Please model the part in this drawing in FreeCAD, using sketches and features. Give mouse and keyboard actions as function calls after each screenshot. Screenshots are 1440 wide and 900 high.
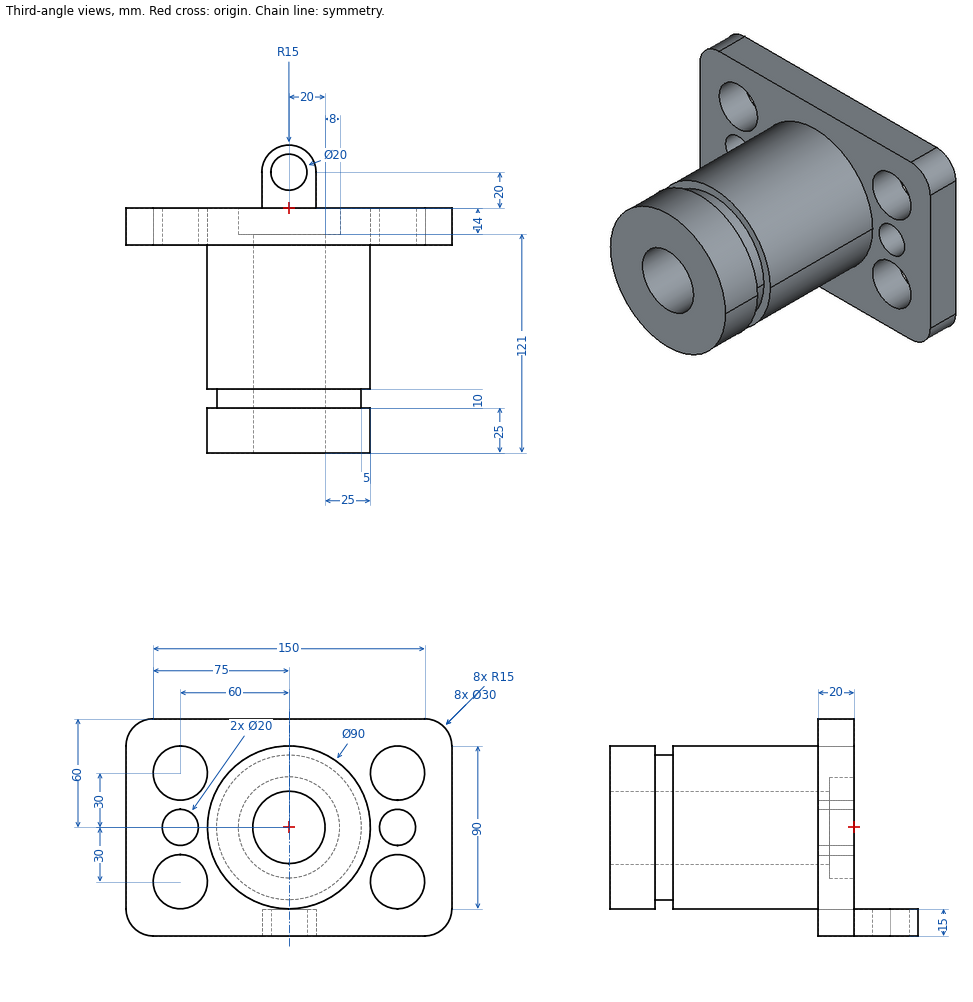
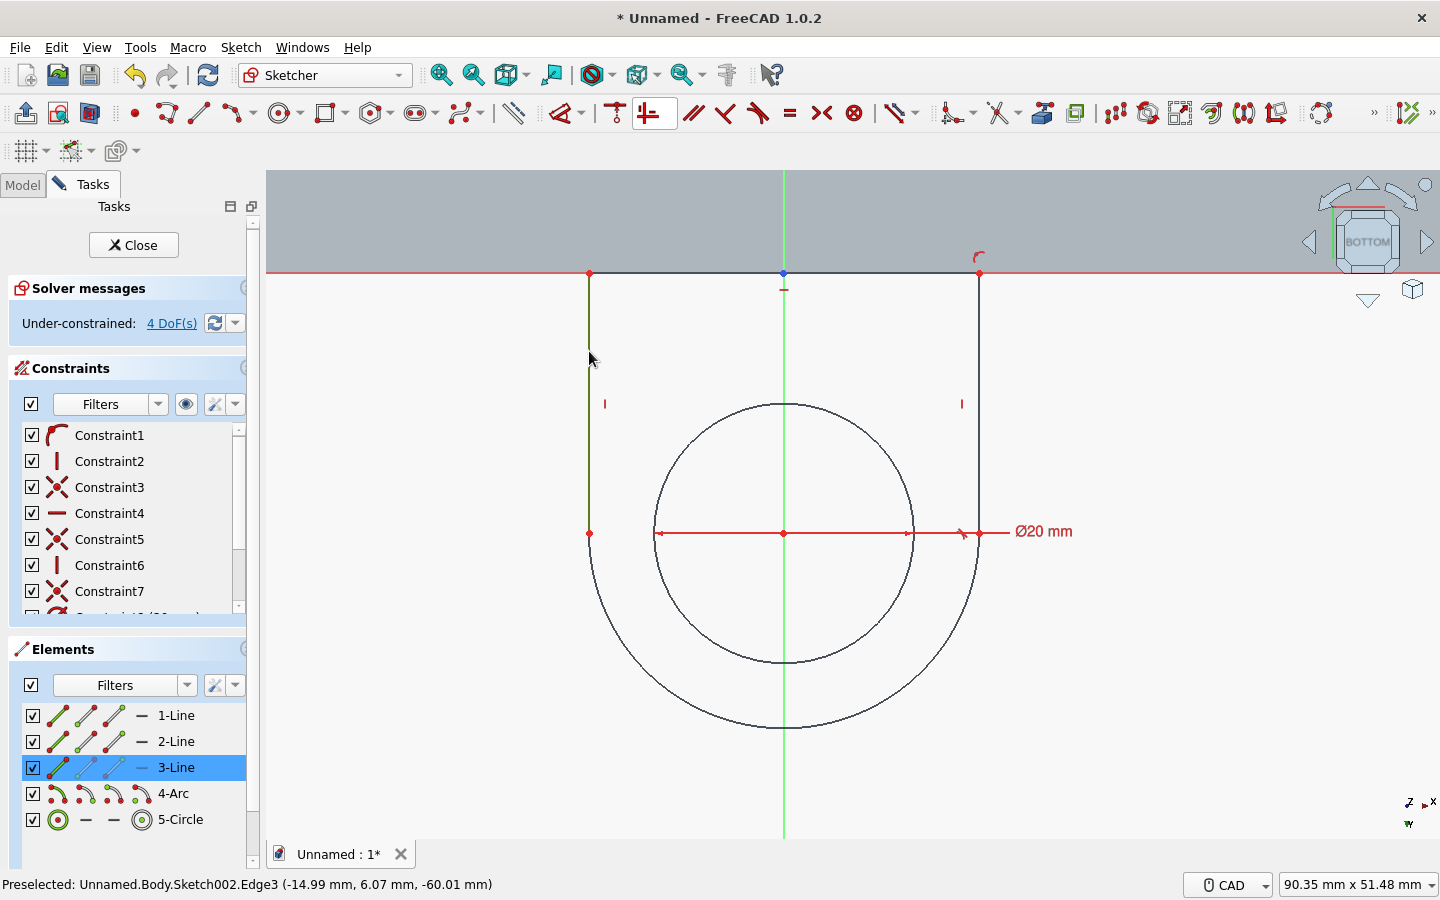
click(670, 691)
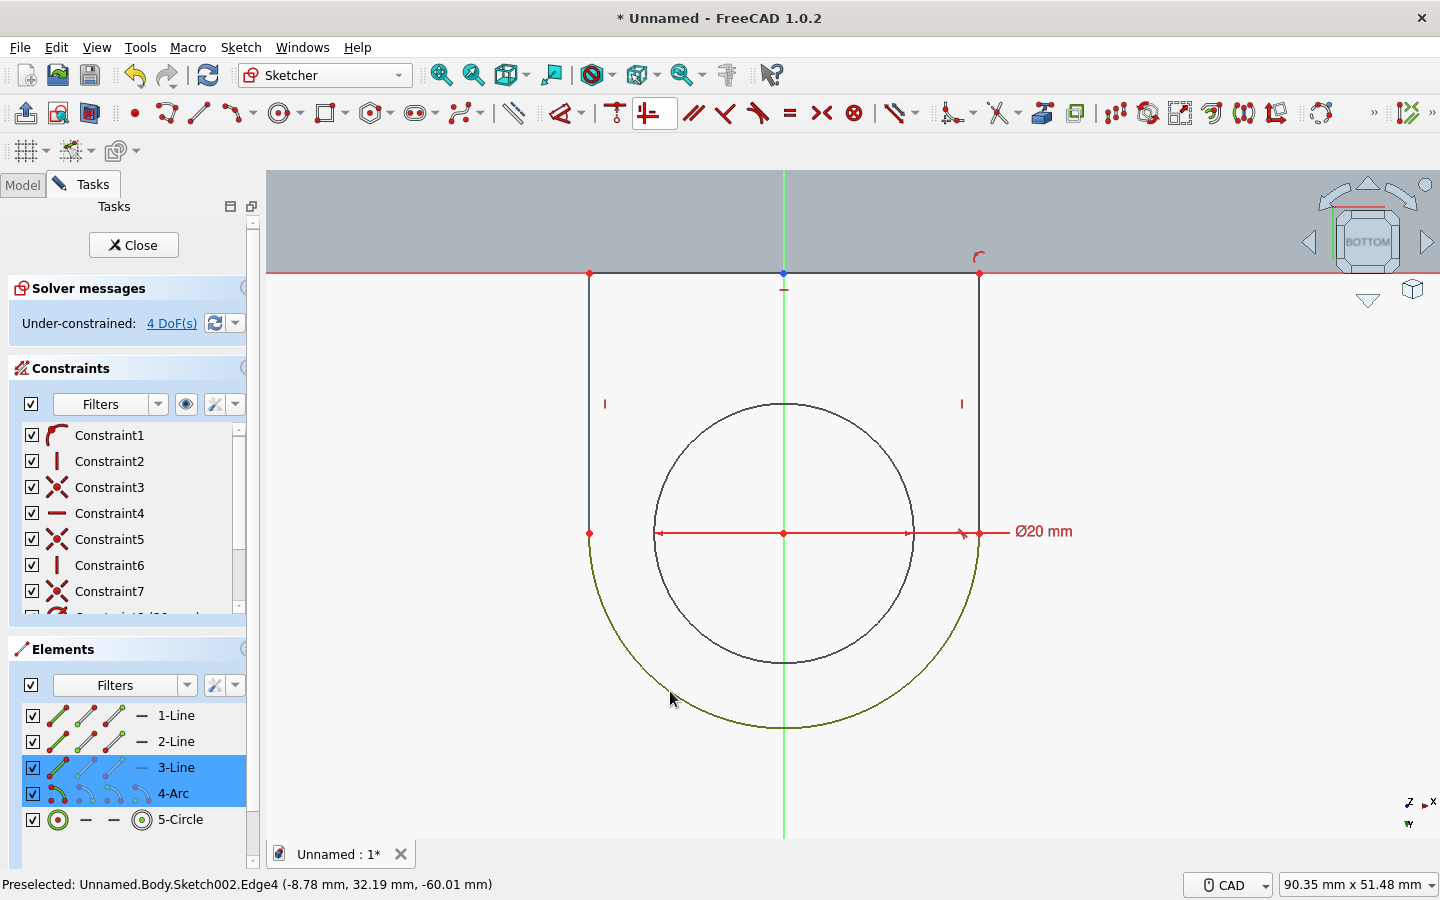
click(758, 114)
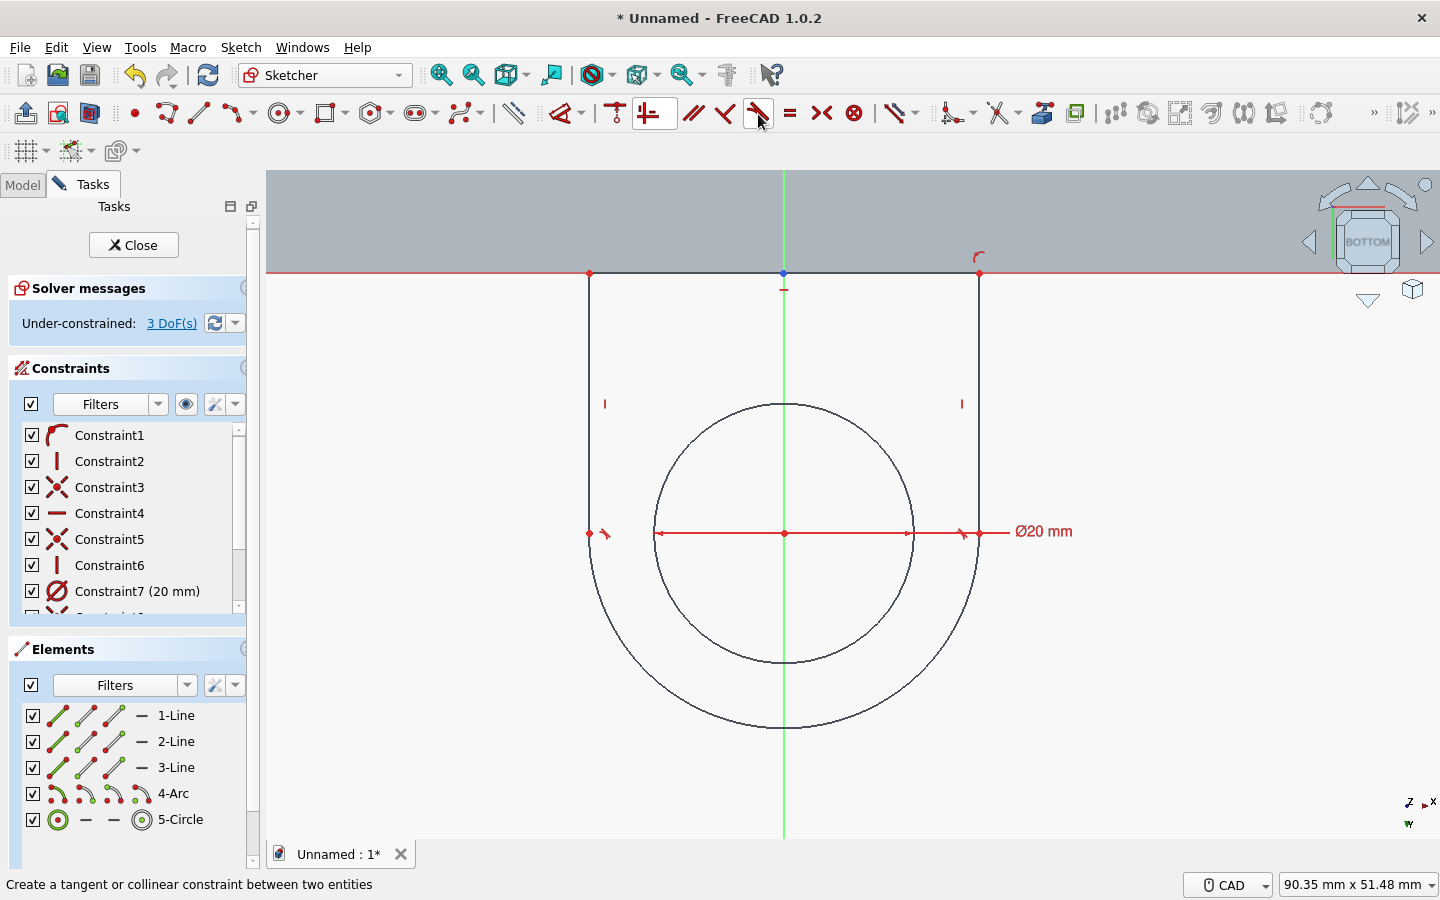
click(784, 533)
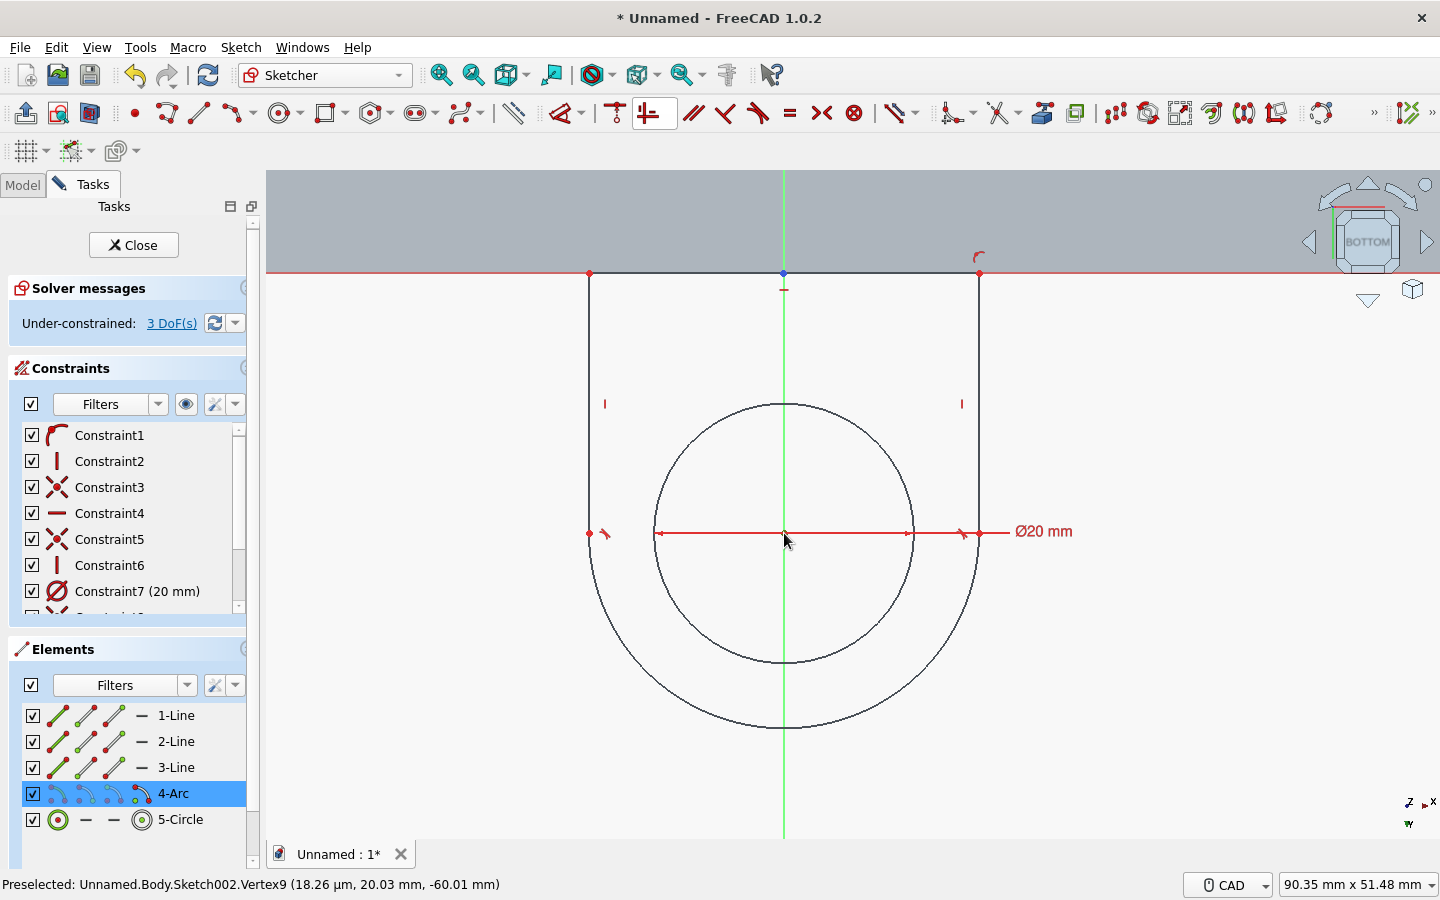
click(784, 767)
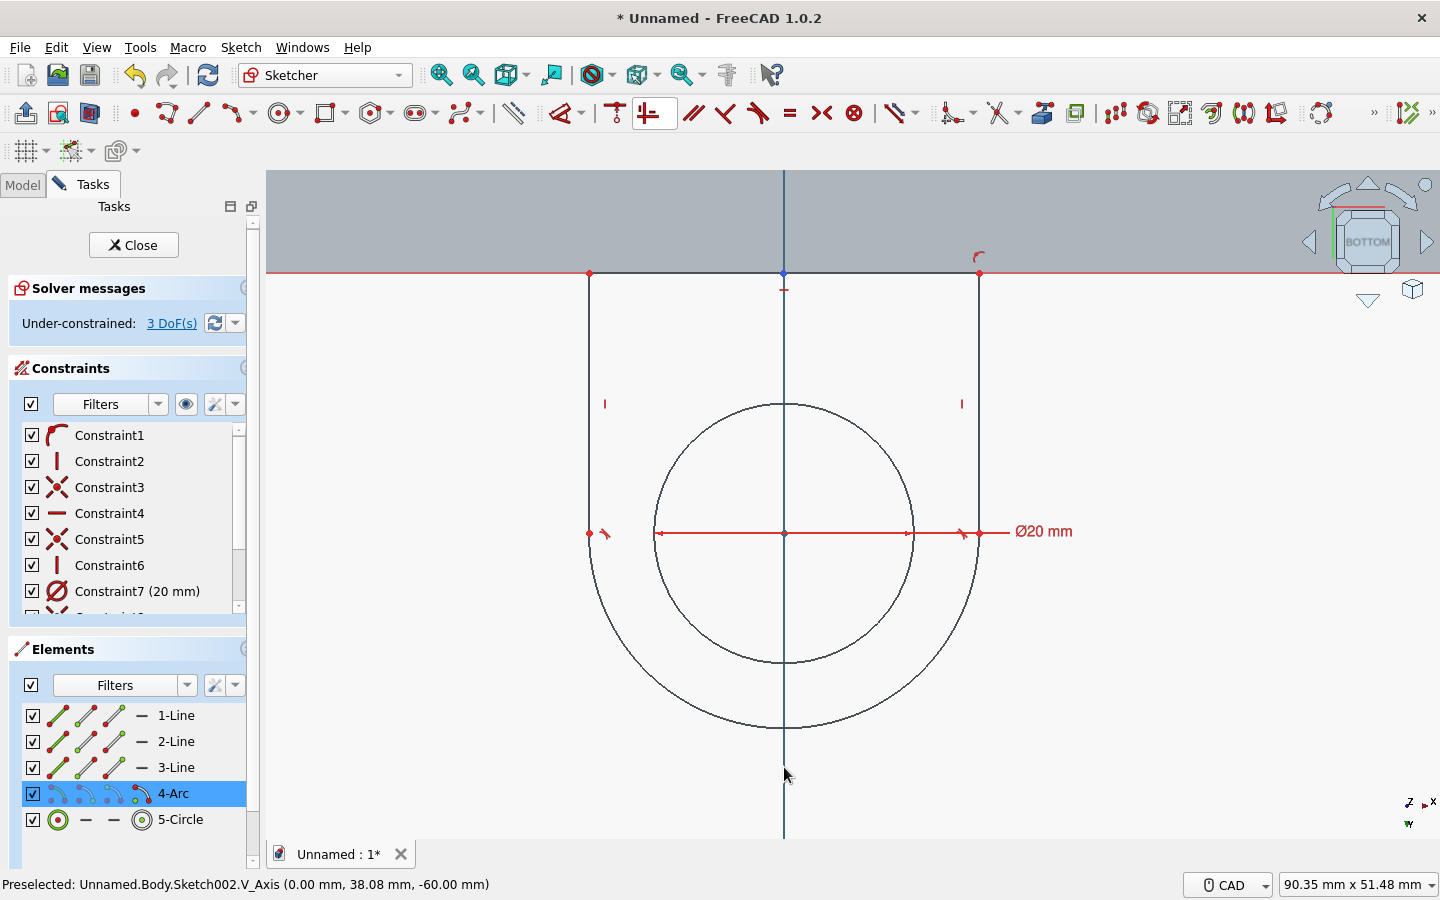
click(616, 114)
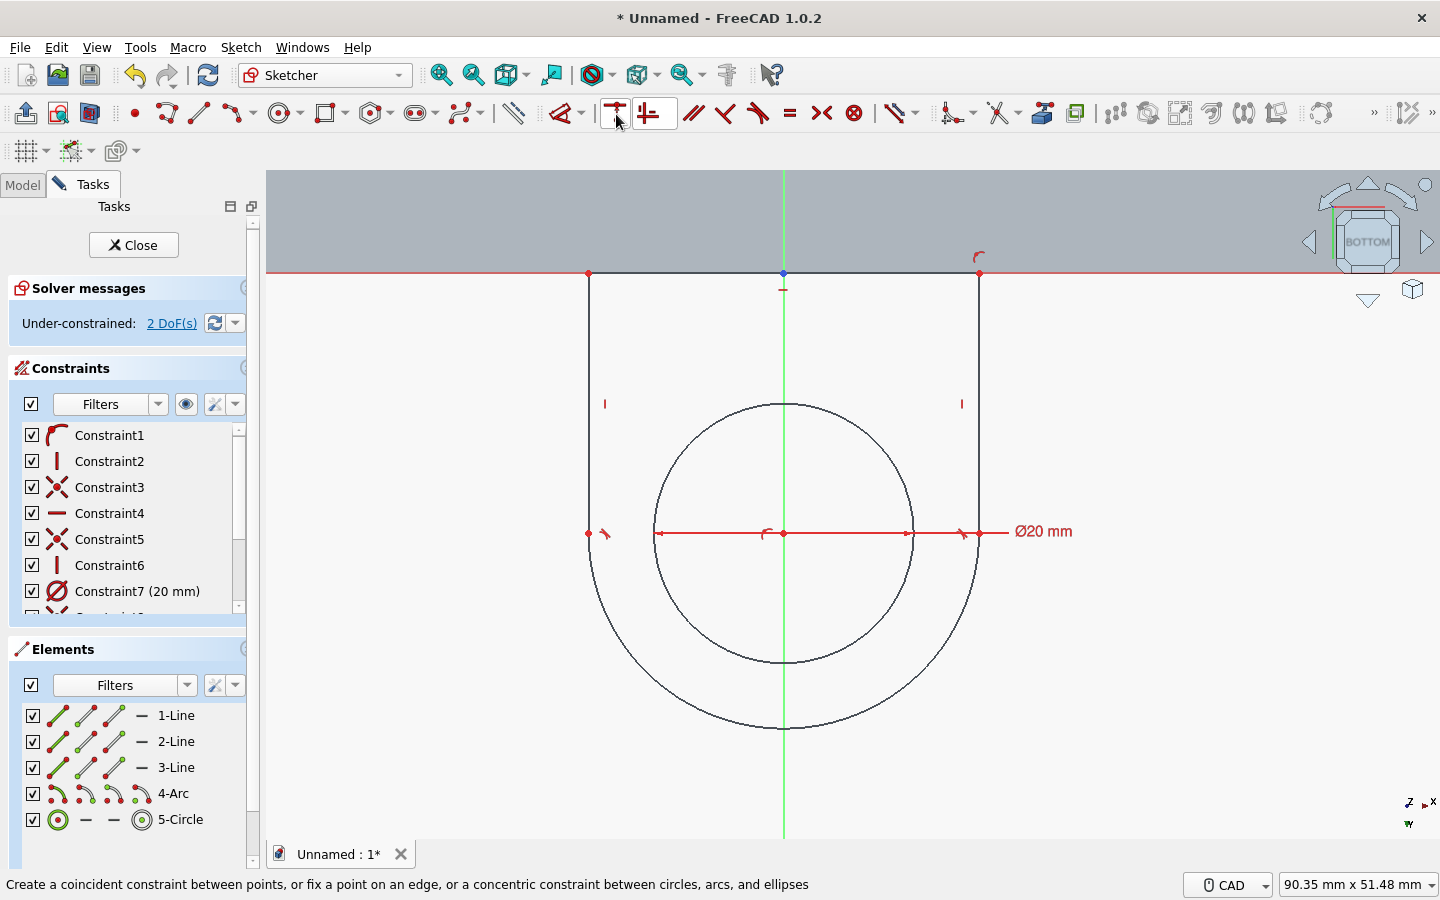
click(560, 114)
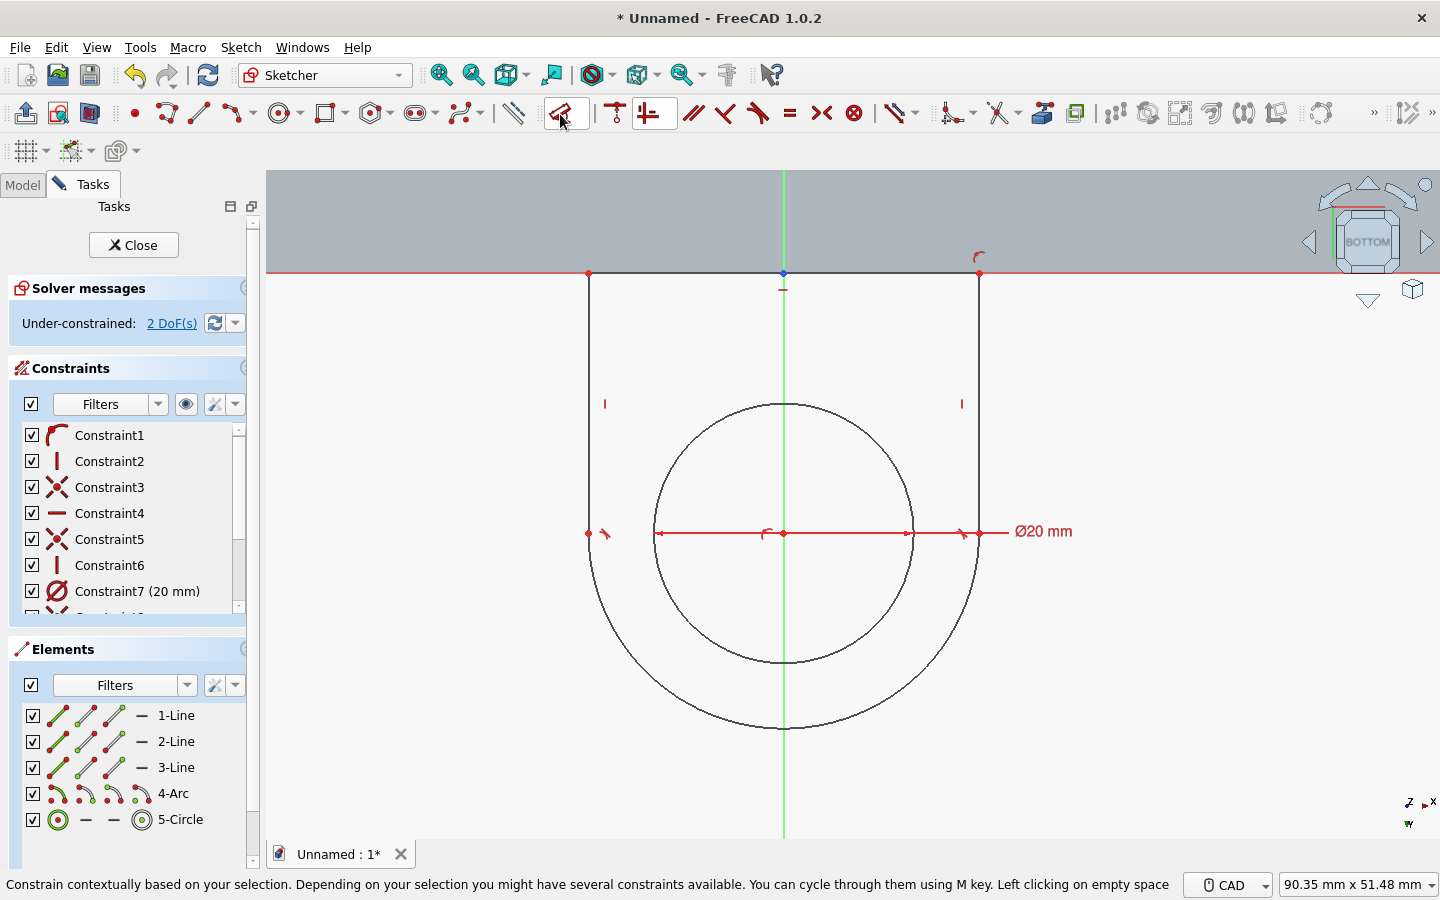
click(669, 691)
click(650, 717)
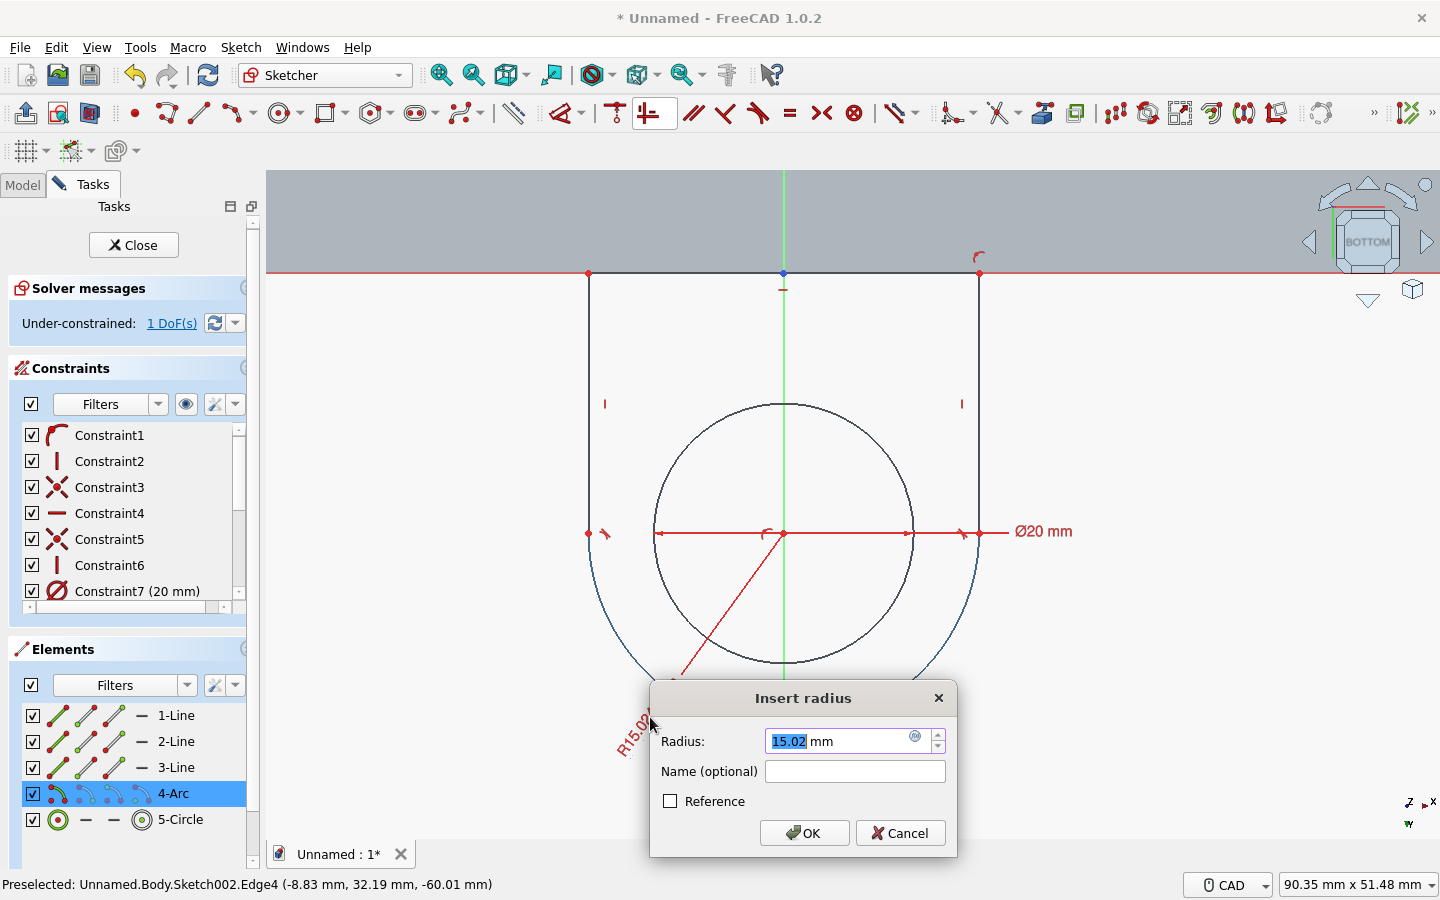
text(15)
key(Return)